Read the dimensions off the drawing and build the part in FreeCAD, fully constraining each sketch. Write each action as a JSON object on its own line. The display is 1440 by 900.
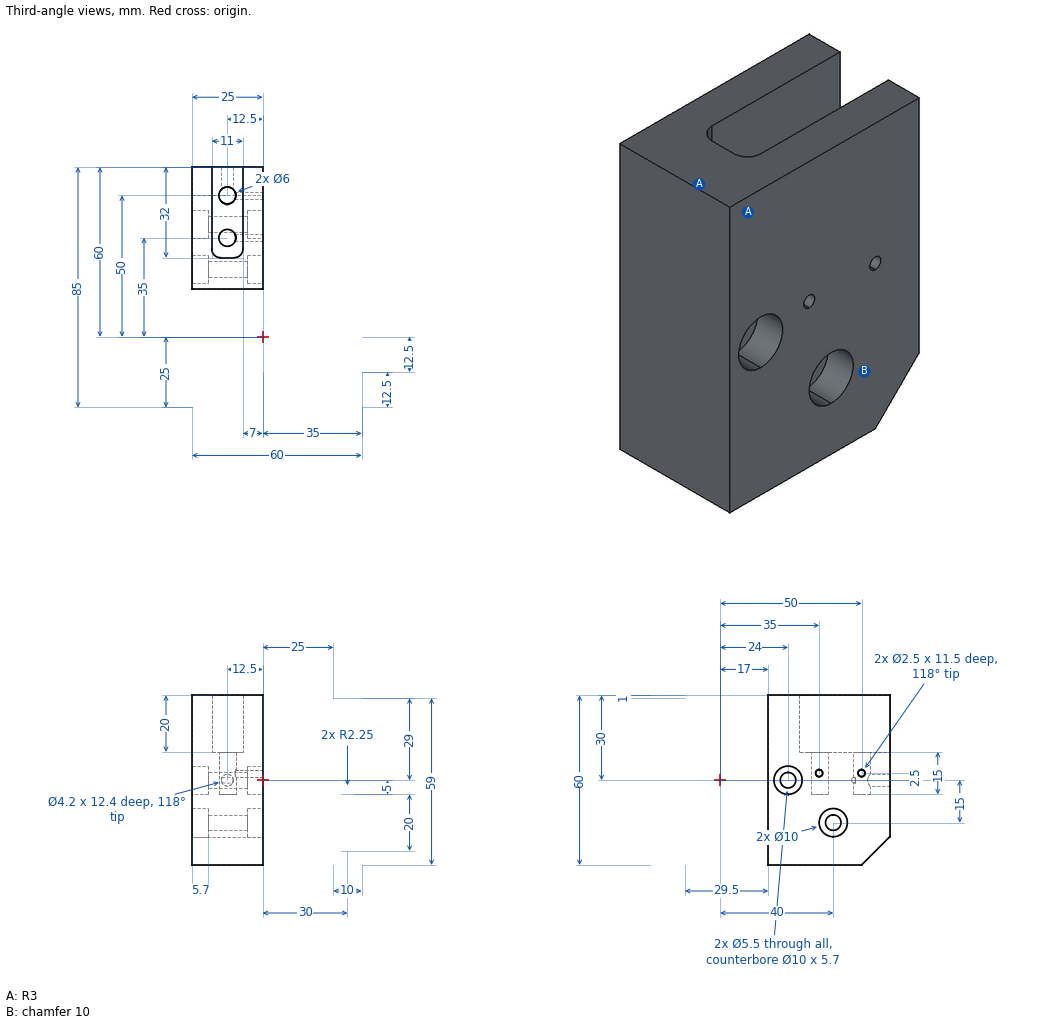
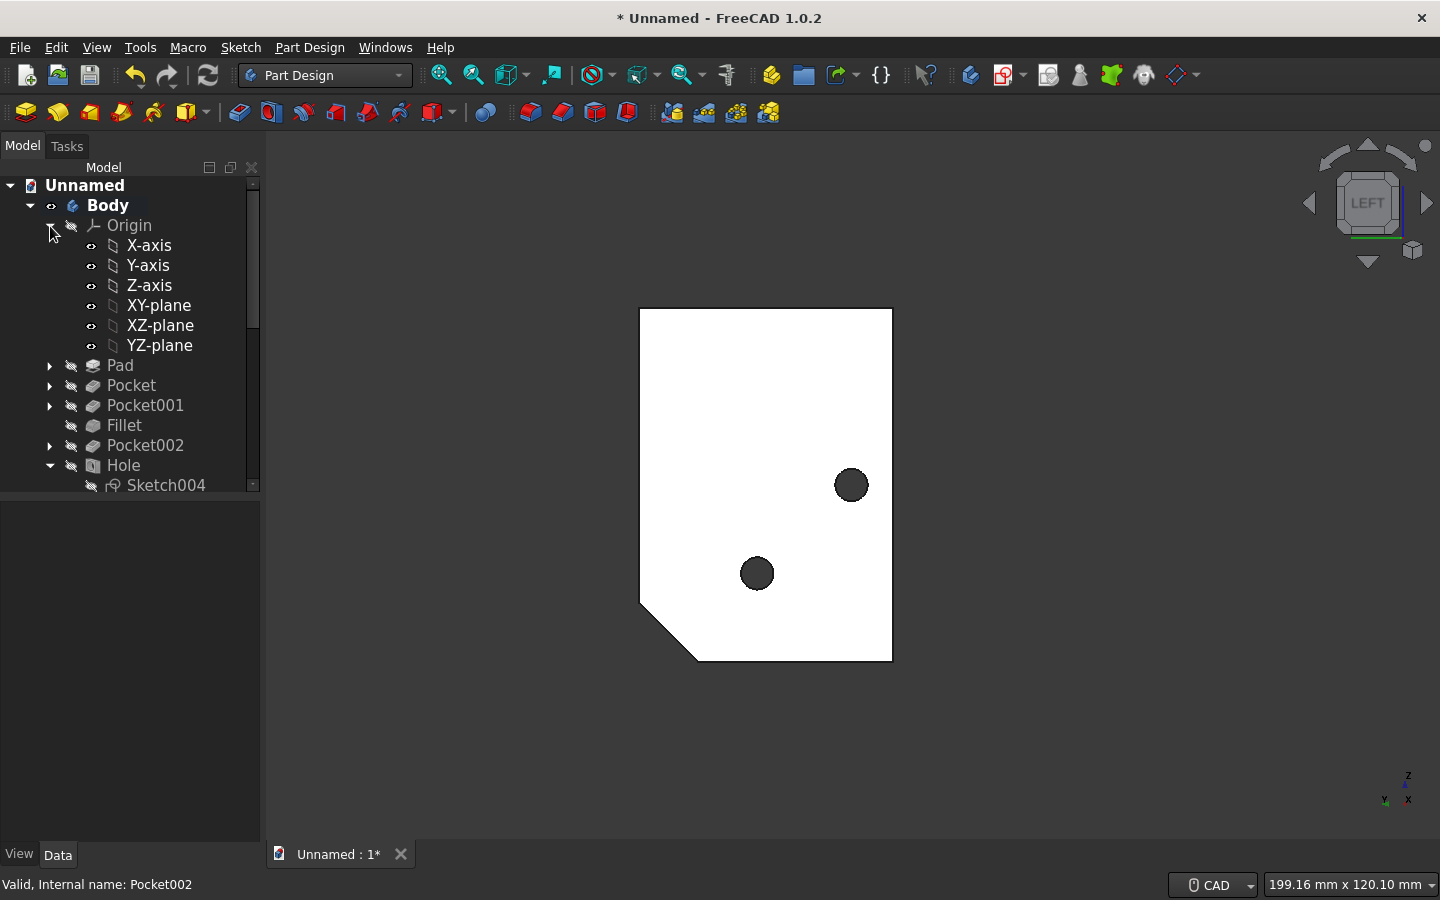
{"action": "left_click", "coordinate": [136, 346]}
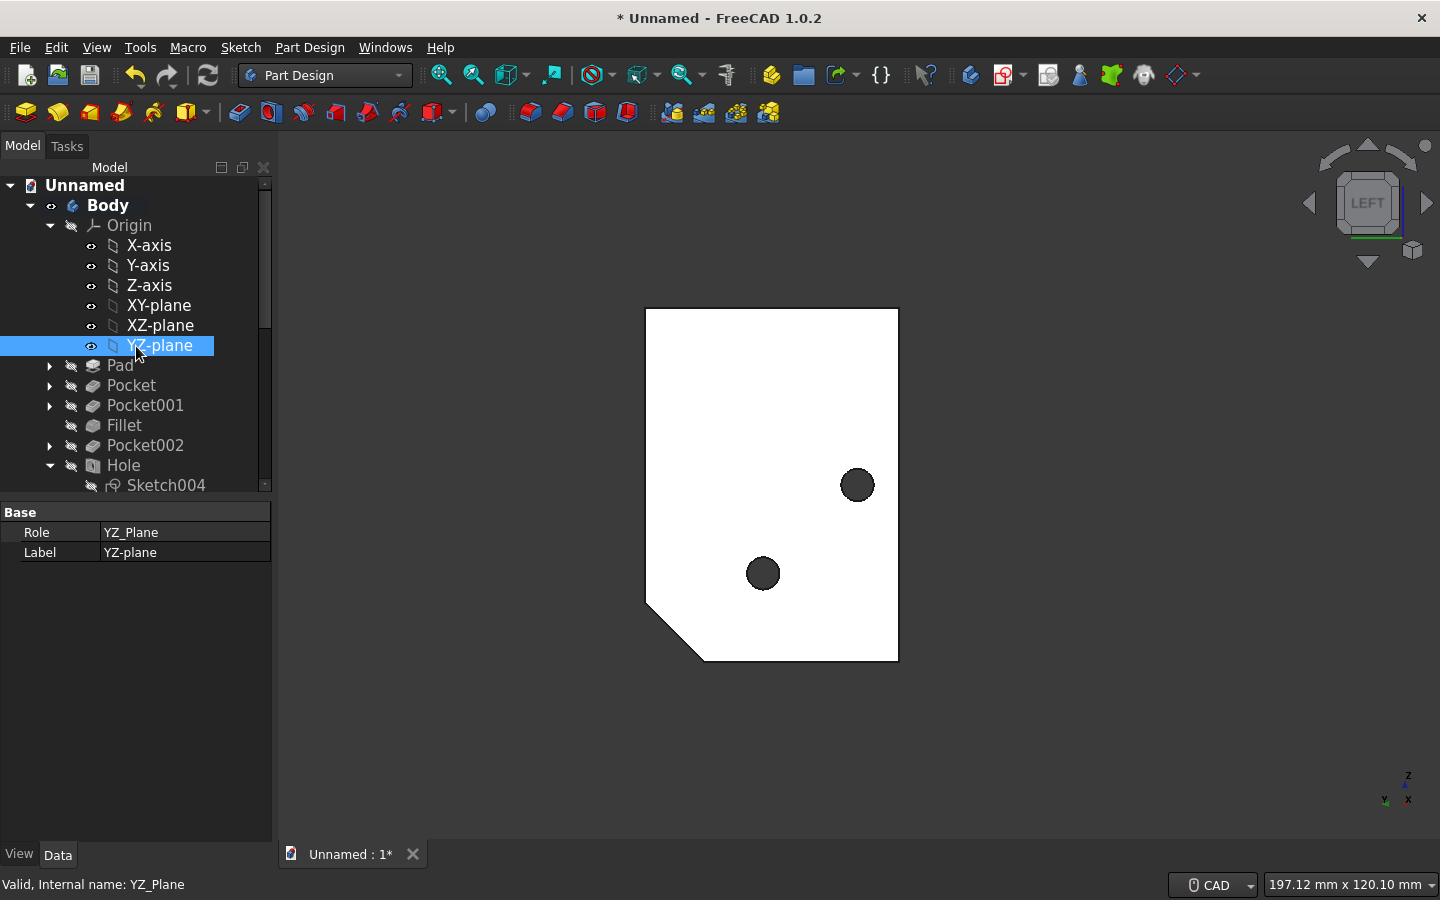
{"action": "left_click", "coordinate": [1176, 76]}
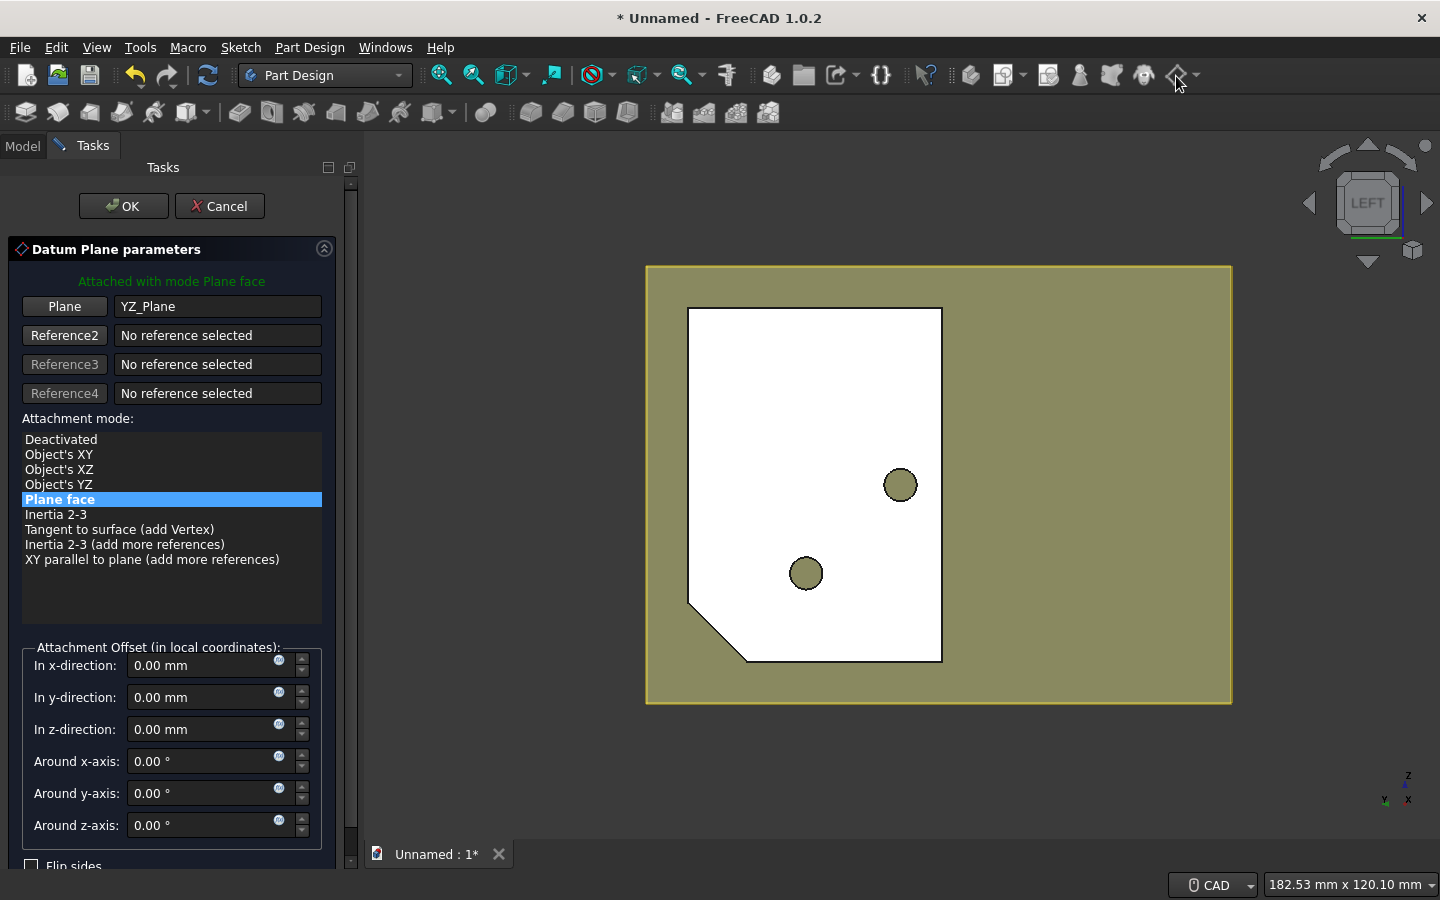
{"action": "triple_click", "coordinate": [210, 729]}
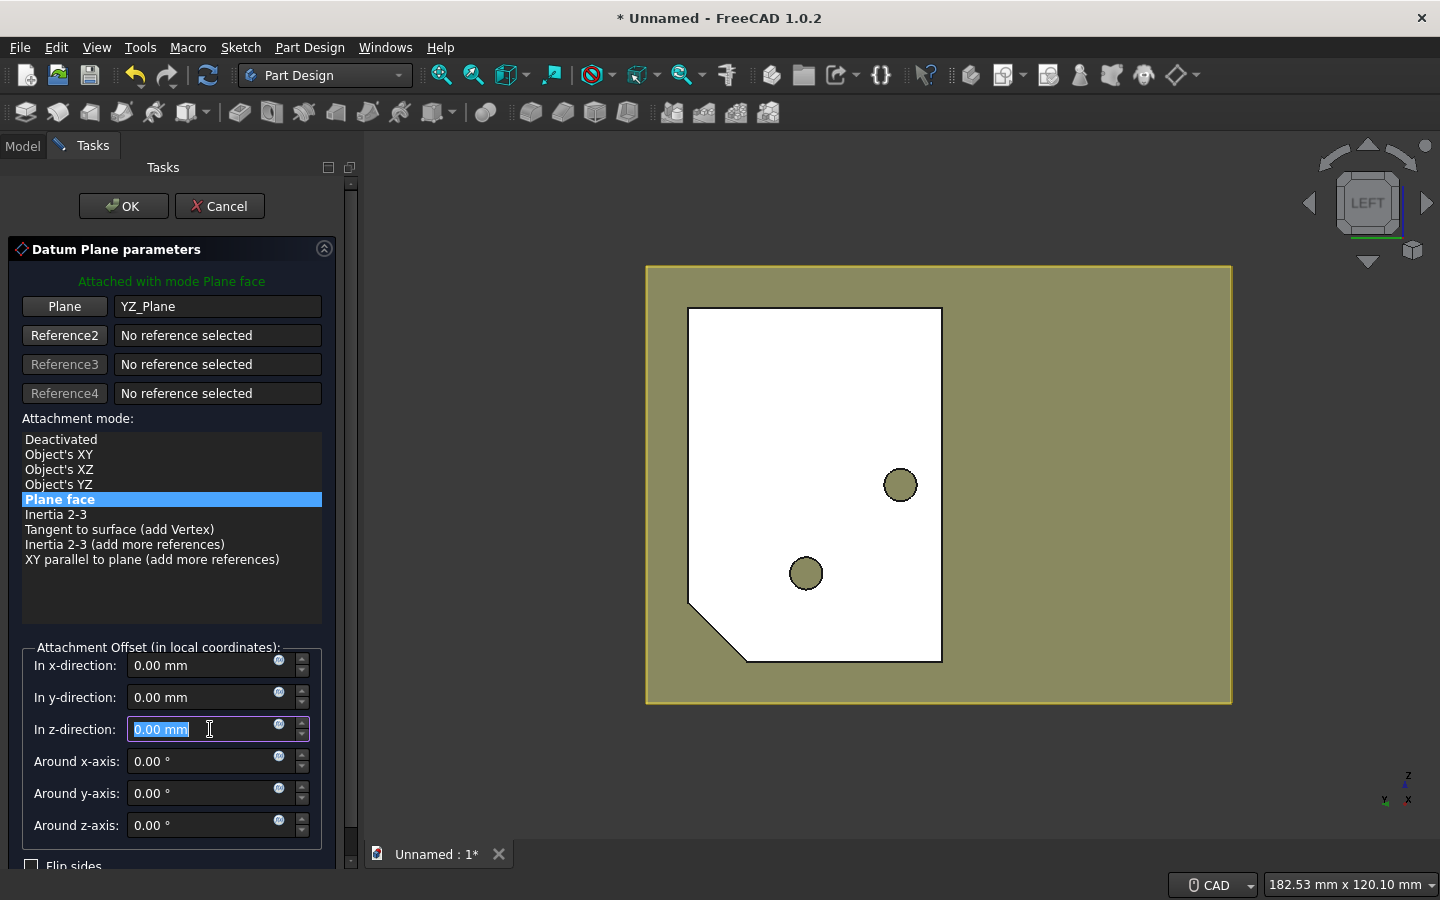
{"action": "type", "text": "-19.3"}
{"action": "key", "text": "Tab"}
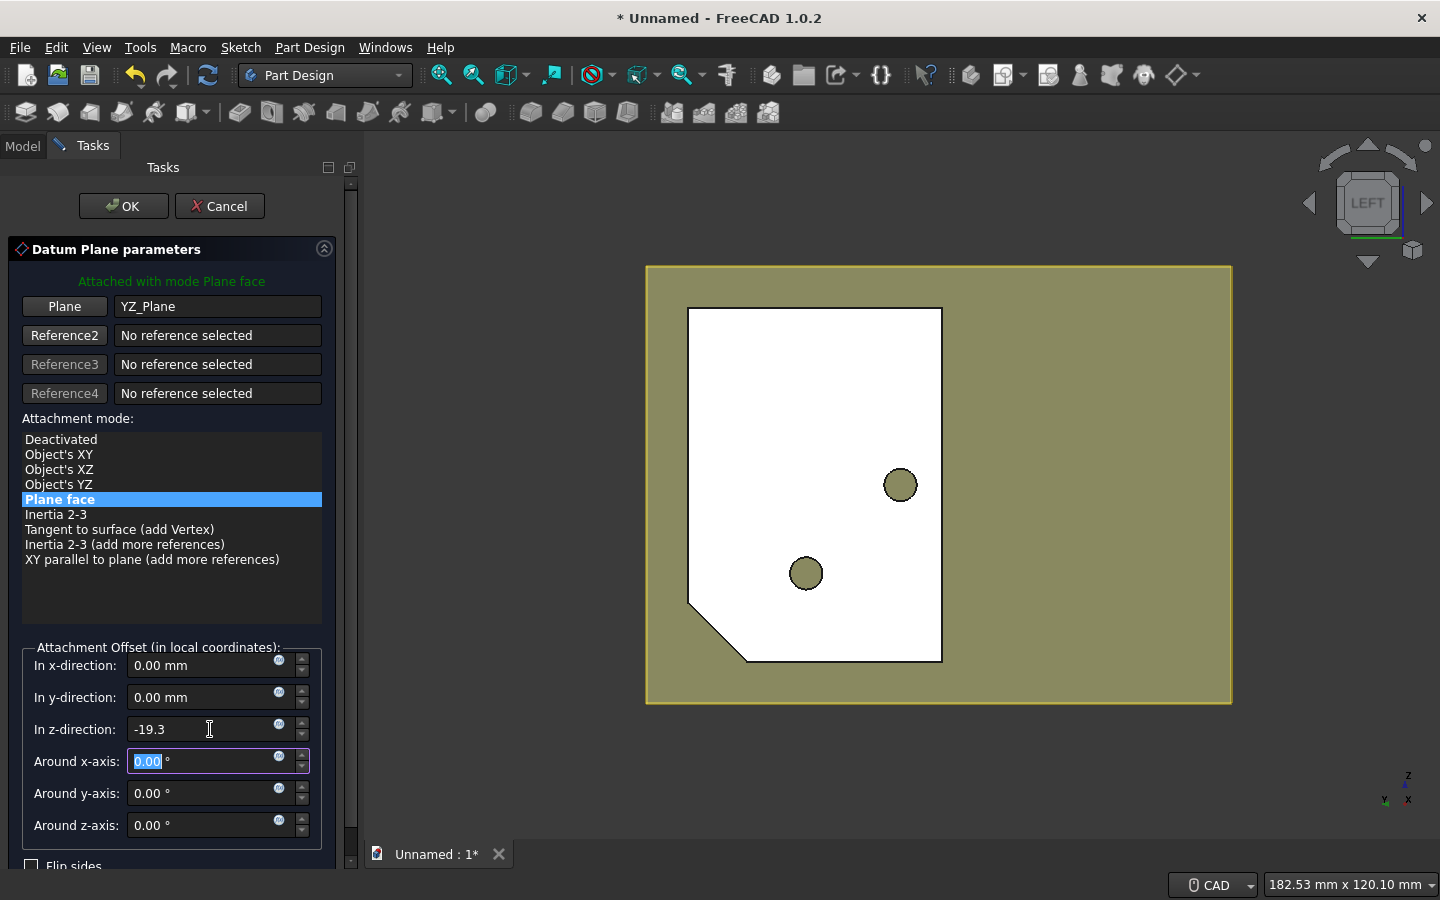
{"action": "left_click", "coordinate": [124, 206]}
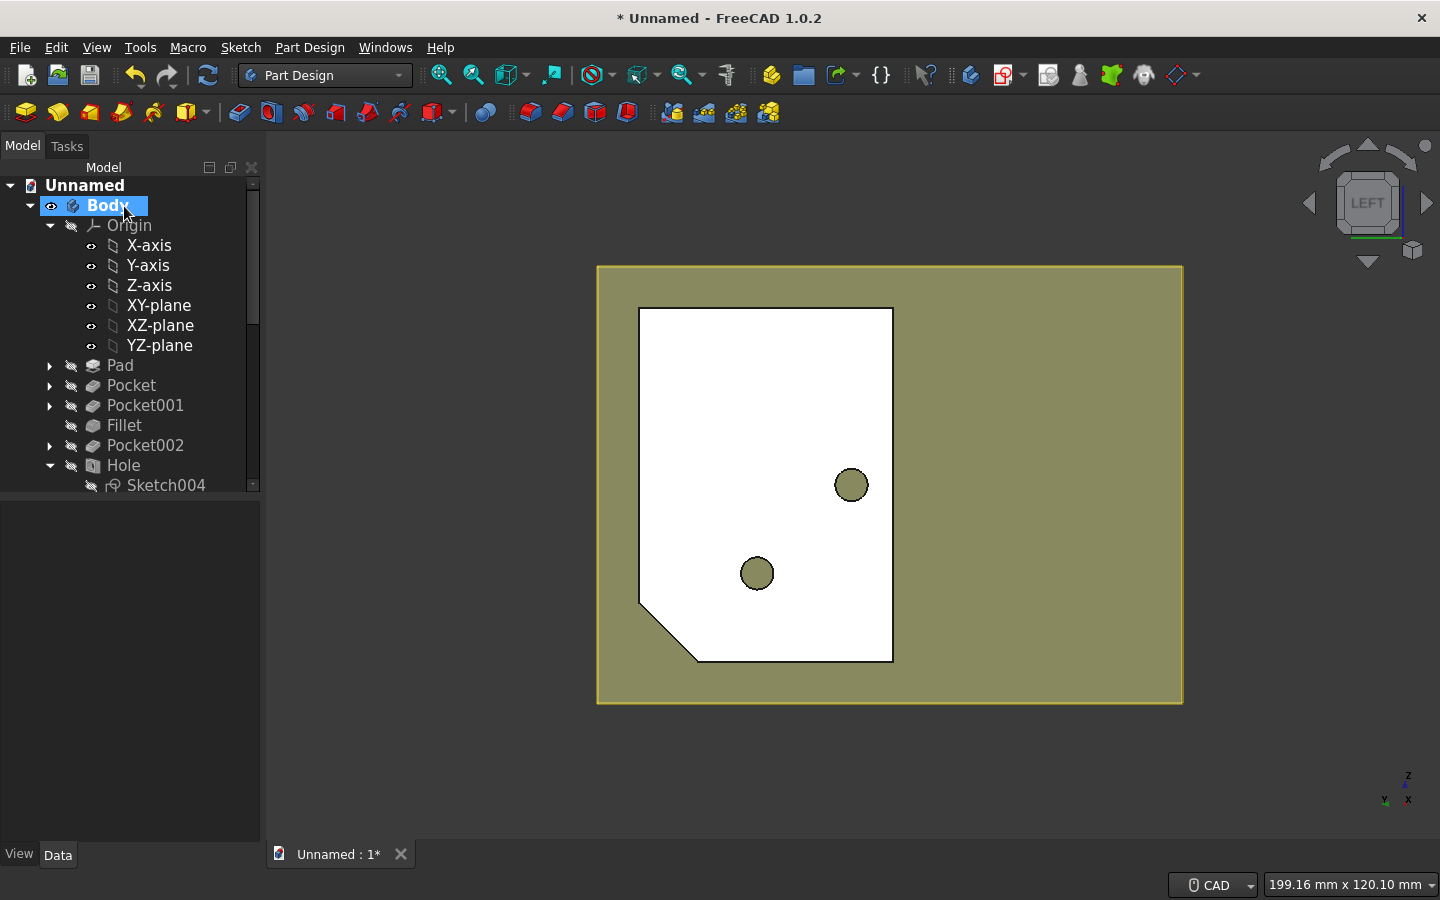
{"action": "scroll", "coordinate": [100, 341], "scroll_direction": "down", "scroll_amount": 3}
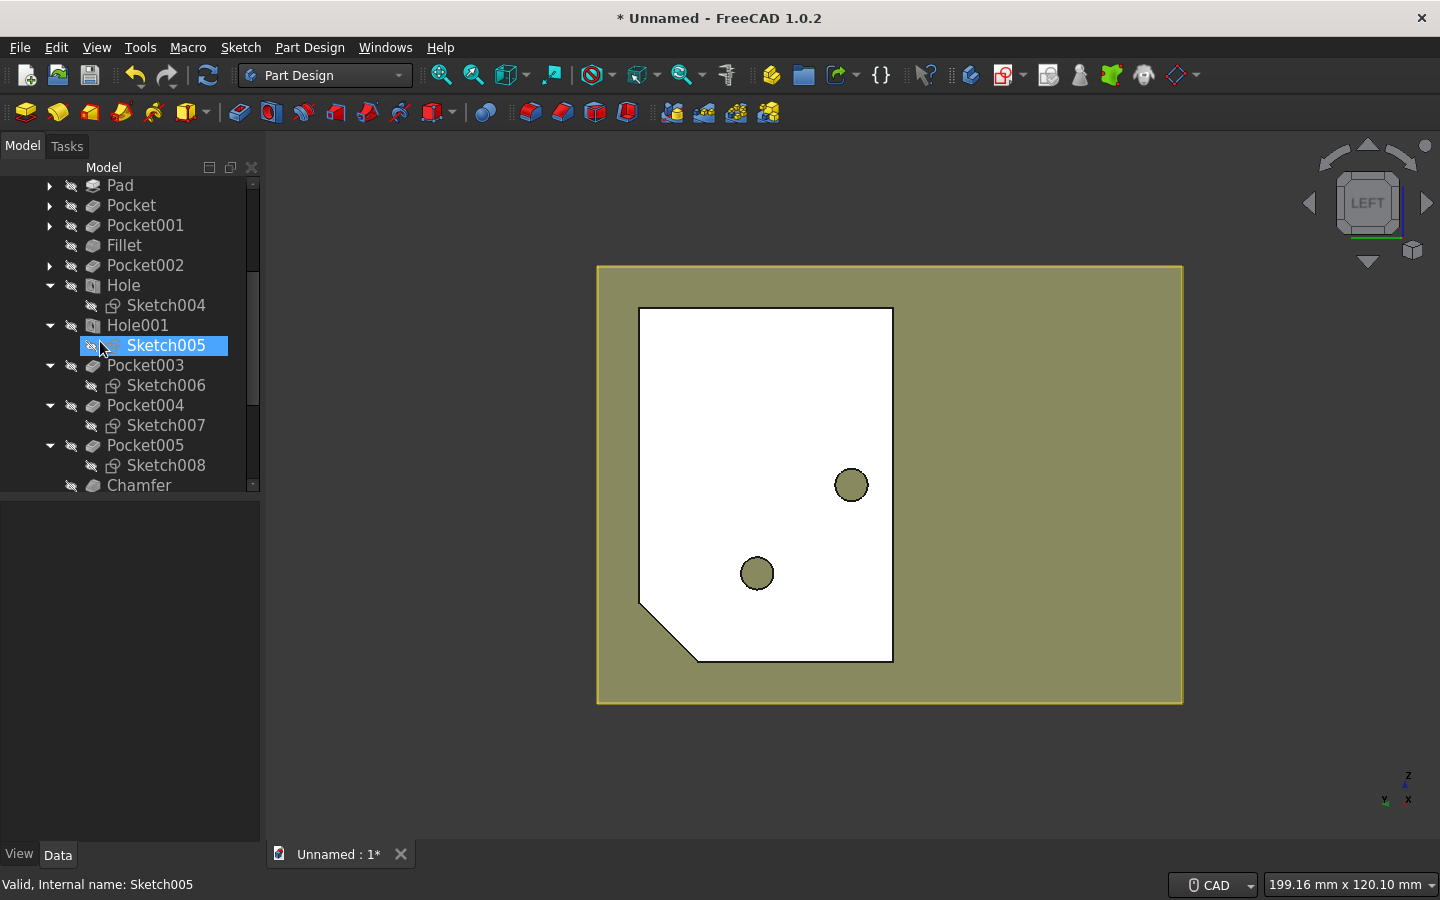
{"action": "scroll", "coordinate": [140, 341], "scroll_direction": "up", "scroll_amount": 15}